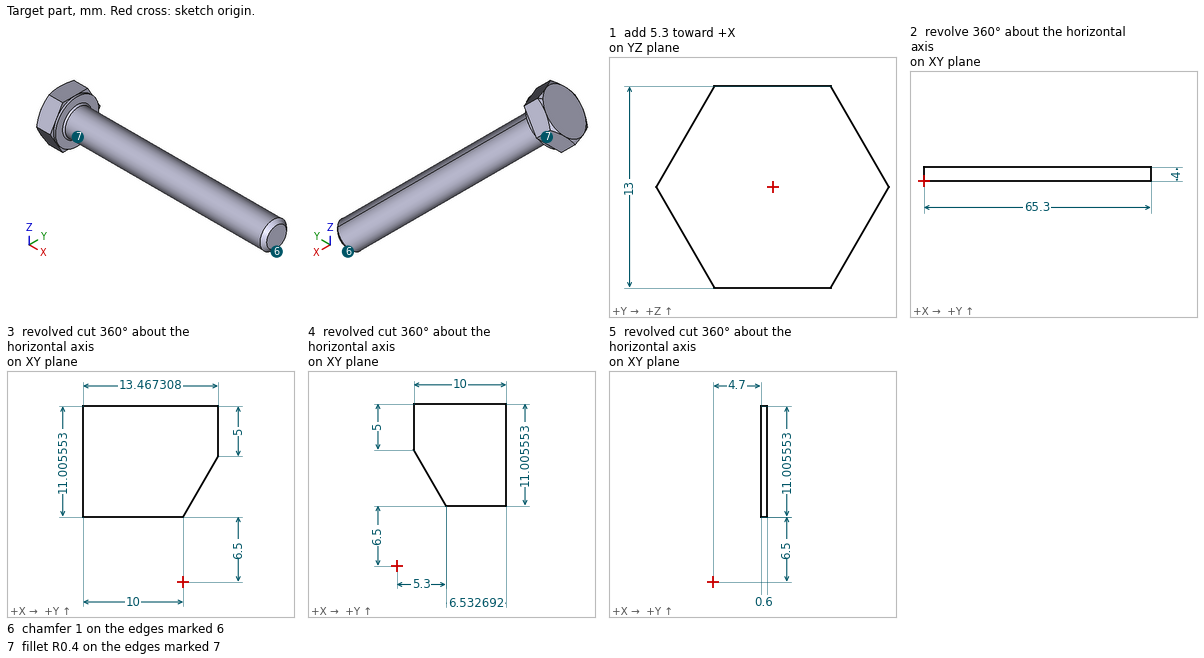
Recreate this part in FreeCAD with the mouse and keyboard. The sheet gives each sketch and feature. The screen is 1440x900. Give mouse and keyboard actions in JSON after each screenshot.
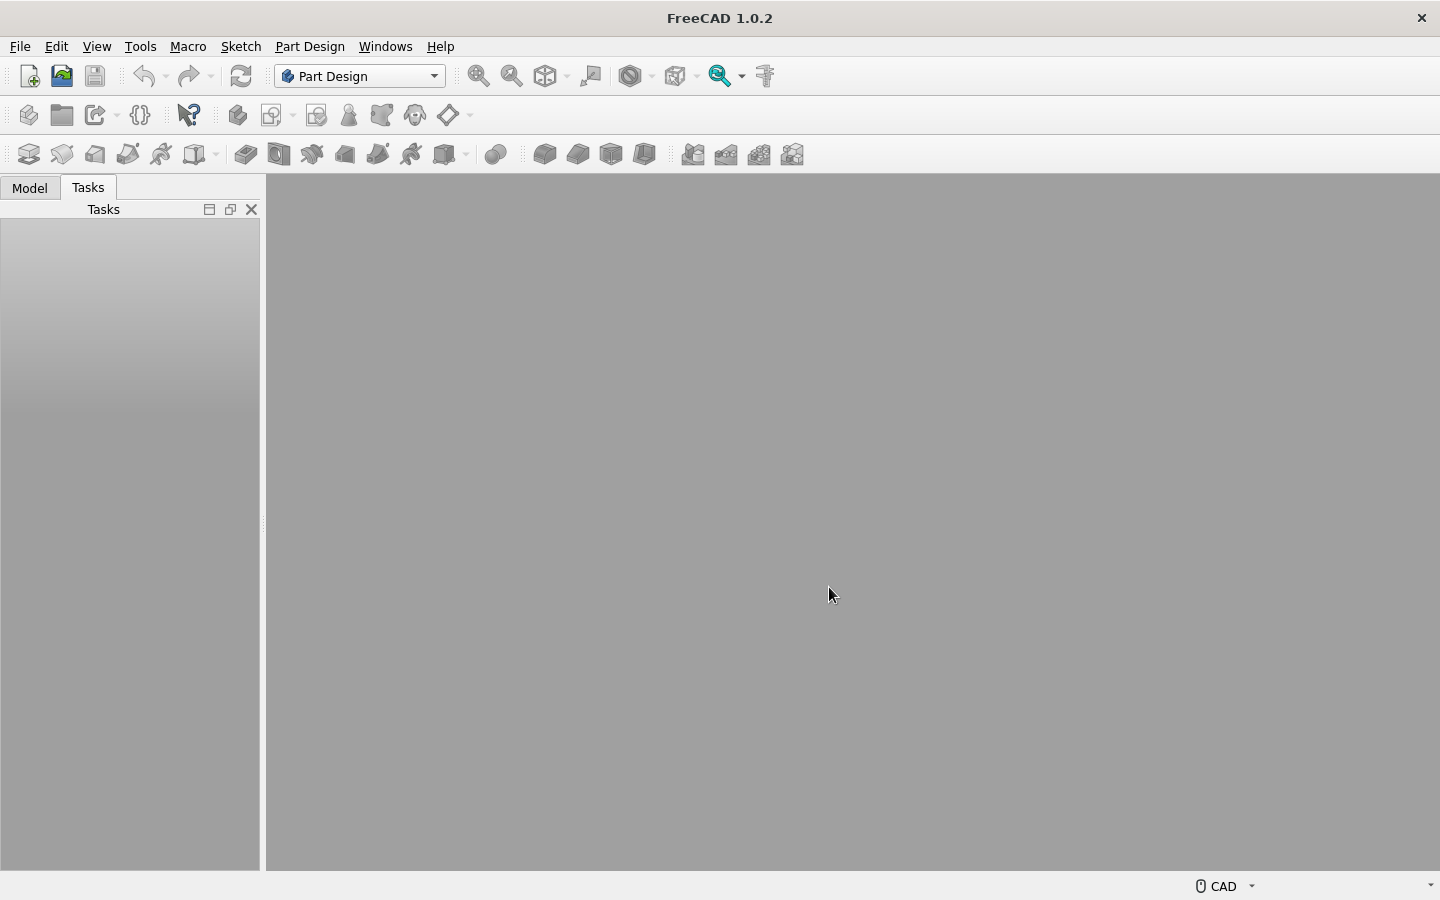
{"action": "left_click", "coordinate": [29, 76]}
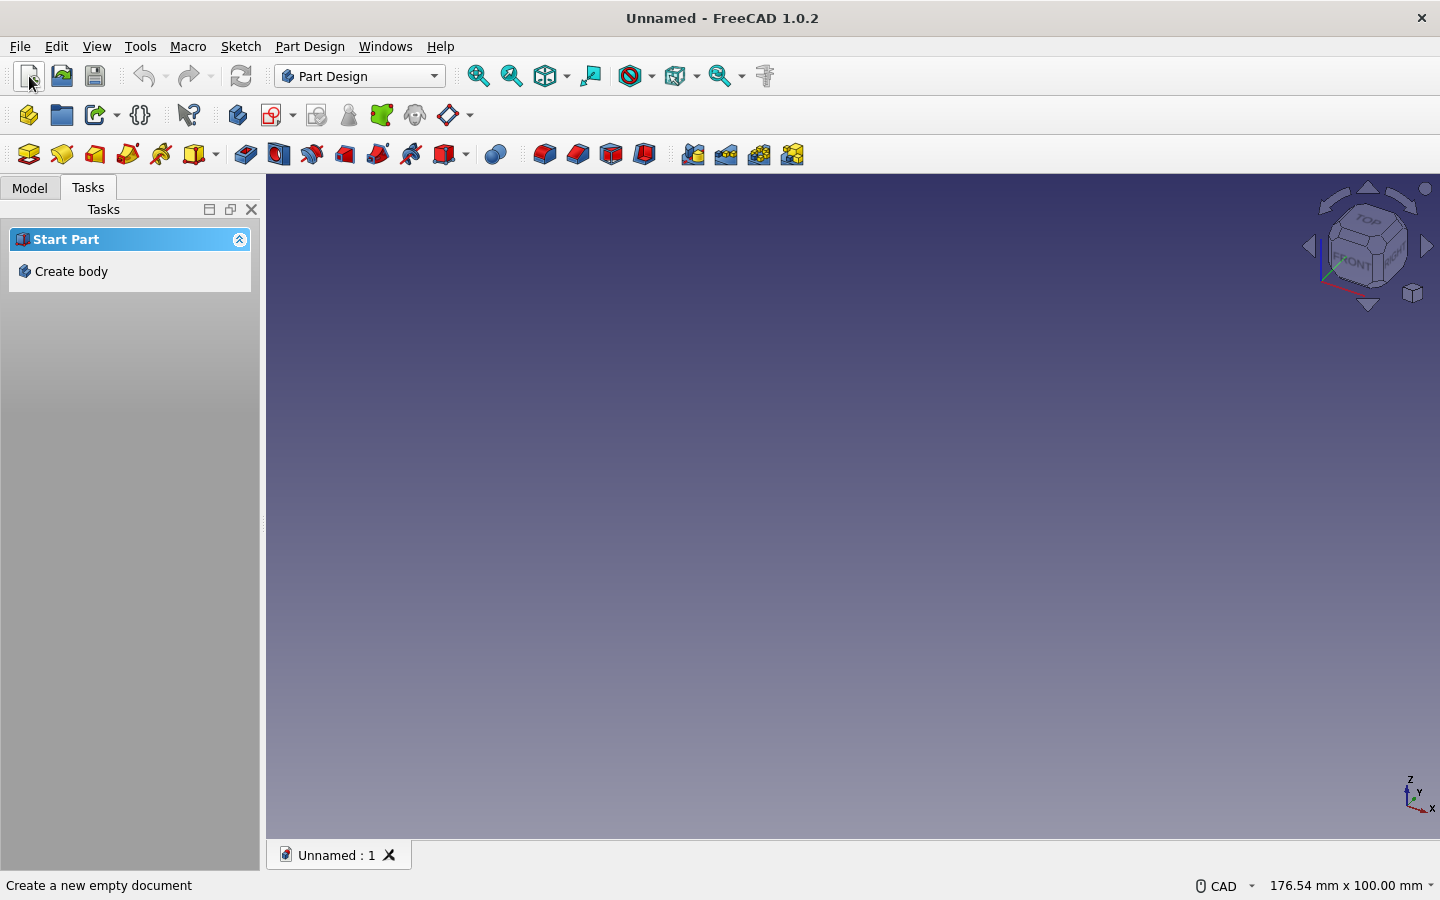
{"action": "left_click", "coordinate": [270, 116]}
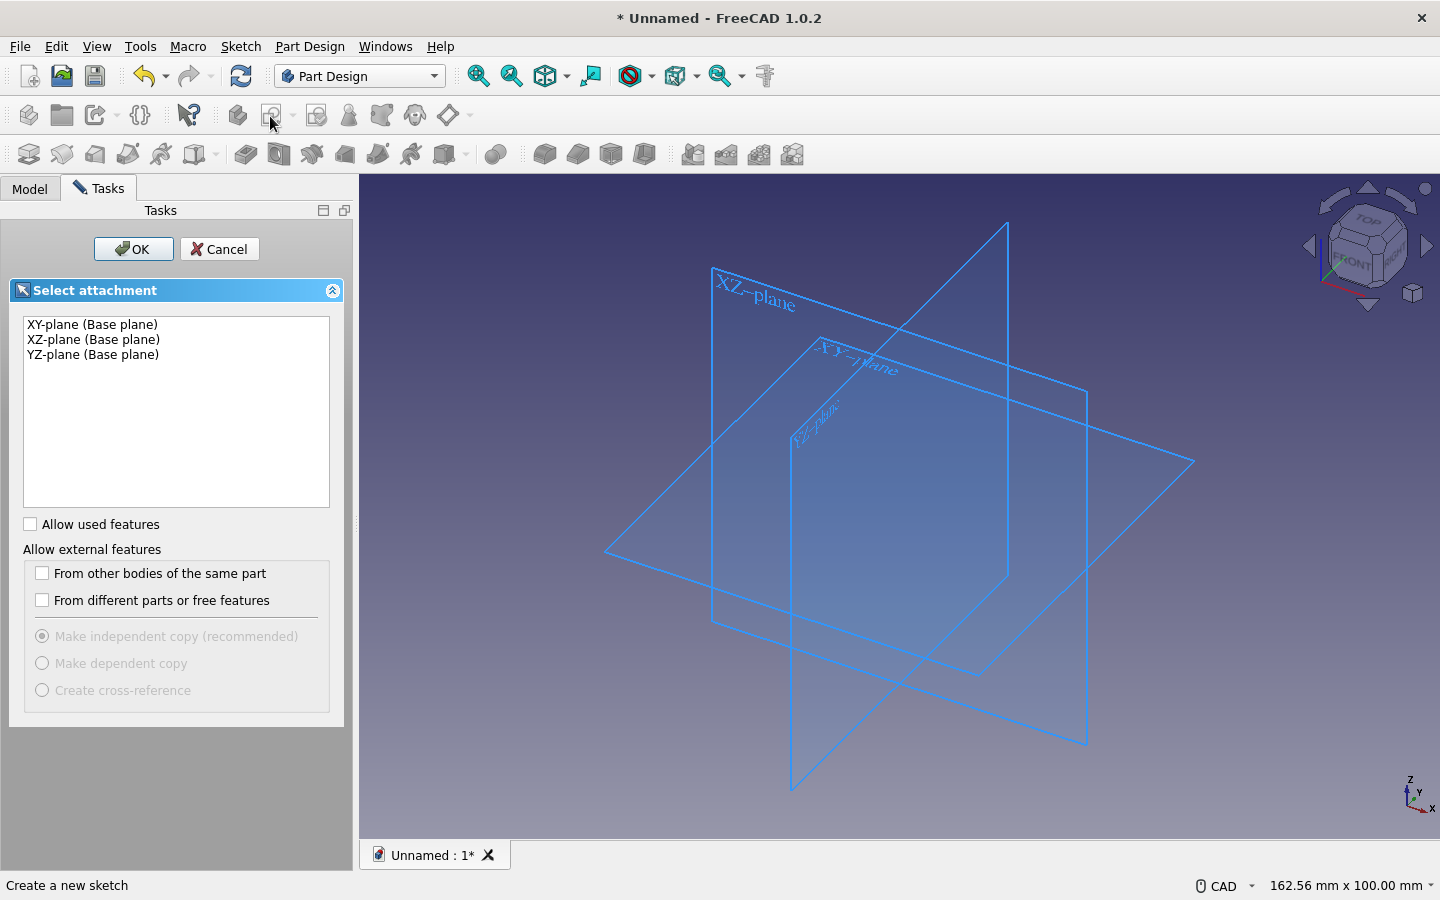
{"action": "left_click", "coordinate": [84, 354]}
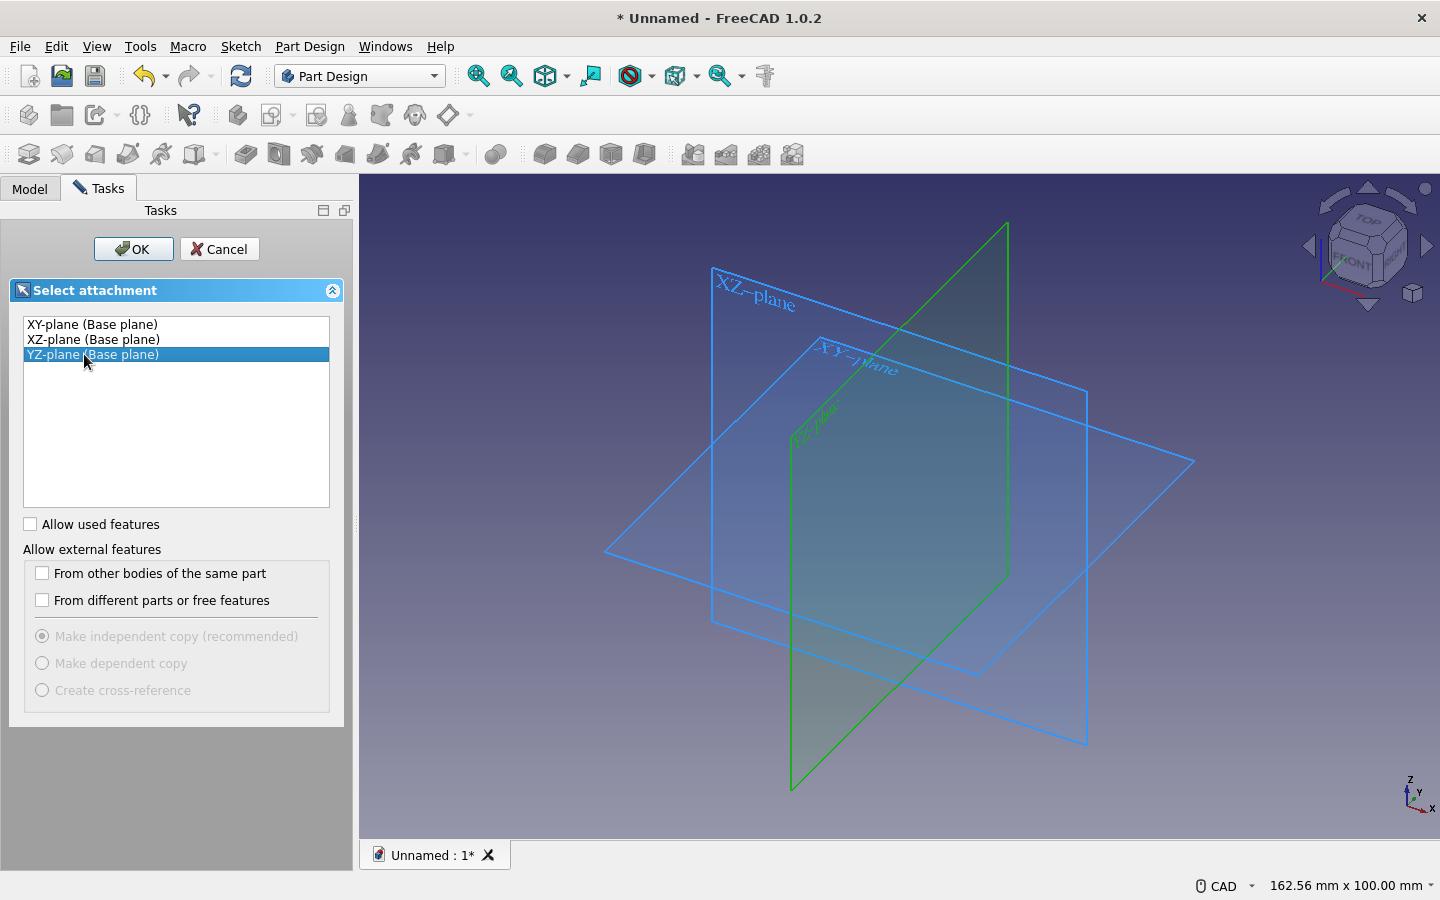
{"action": "left_click", "coordinate": [134, 249]}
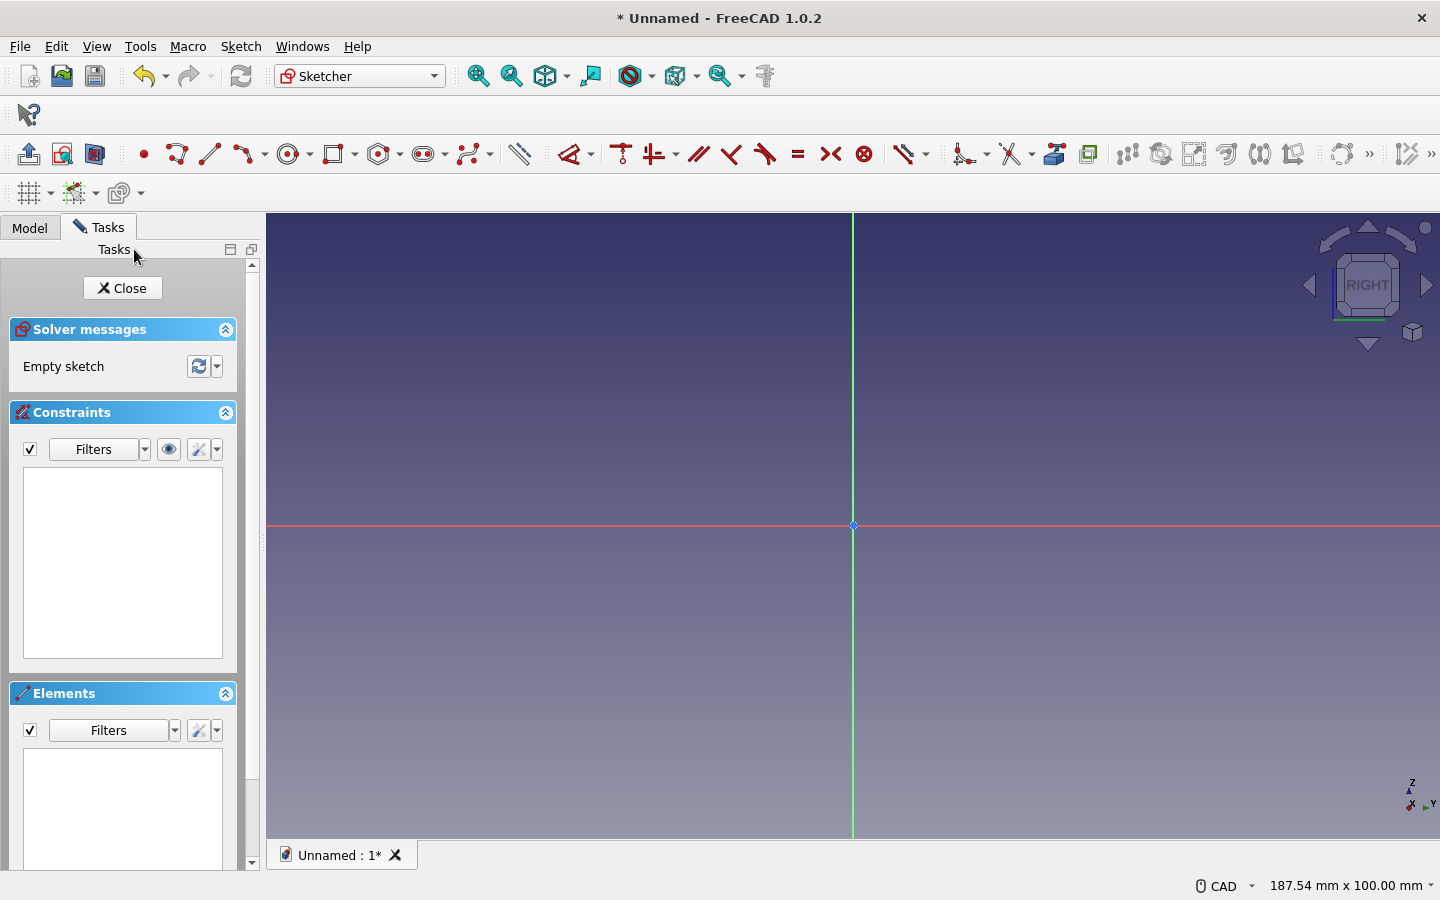
{"action": "scroll", "coordinate": [870, 526], "scroll_direction": "up", "scroll_amount": 8}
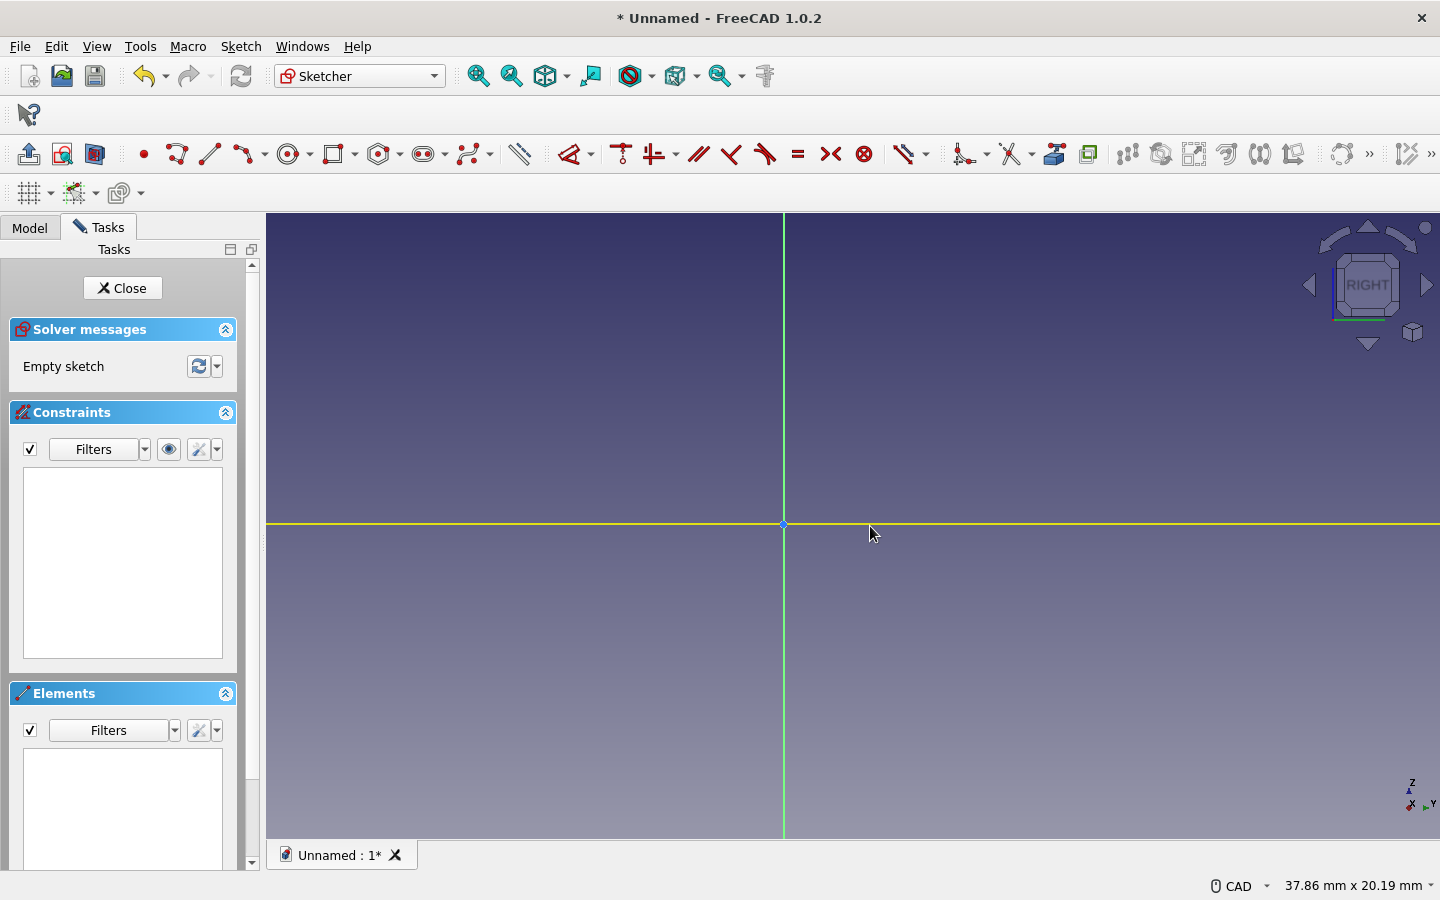
{"action": "left_click", "coordinate": [378, 154]}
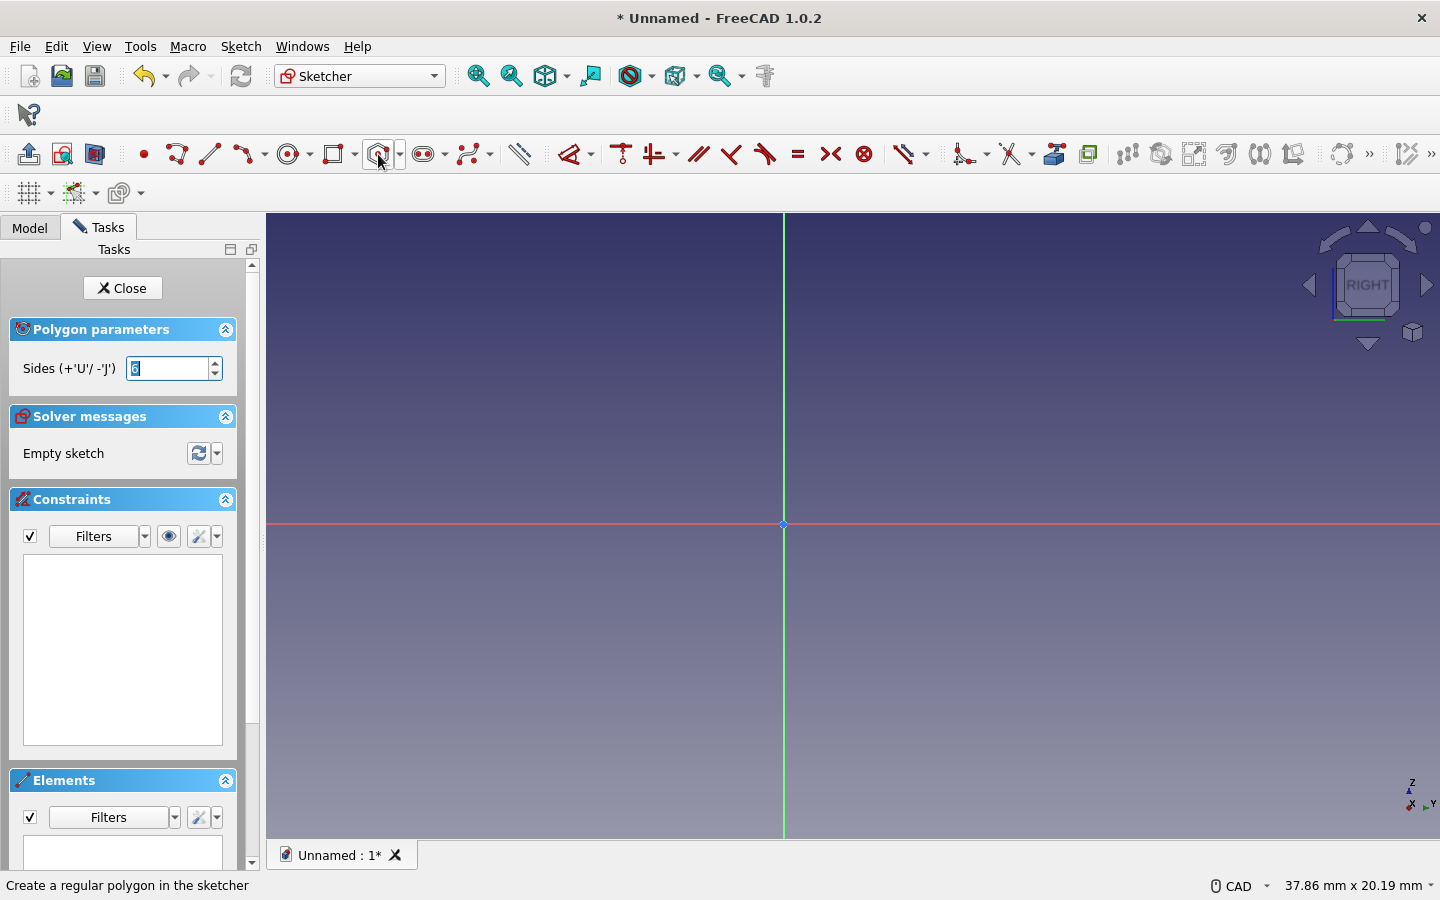
{"action": "left_click", "coordinate": [784, 524]}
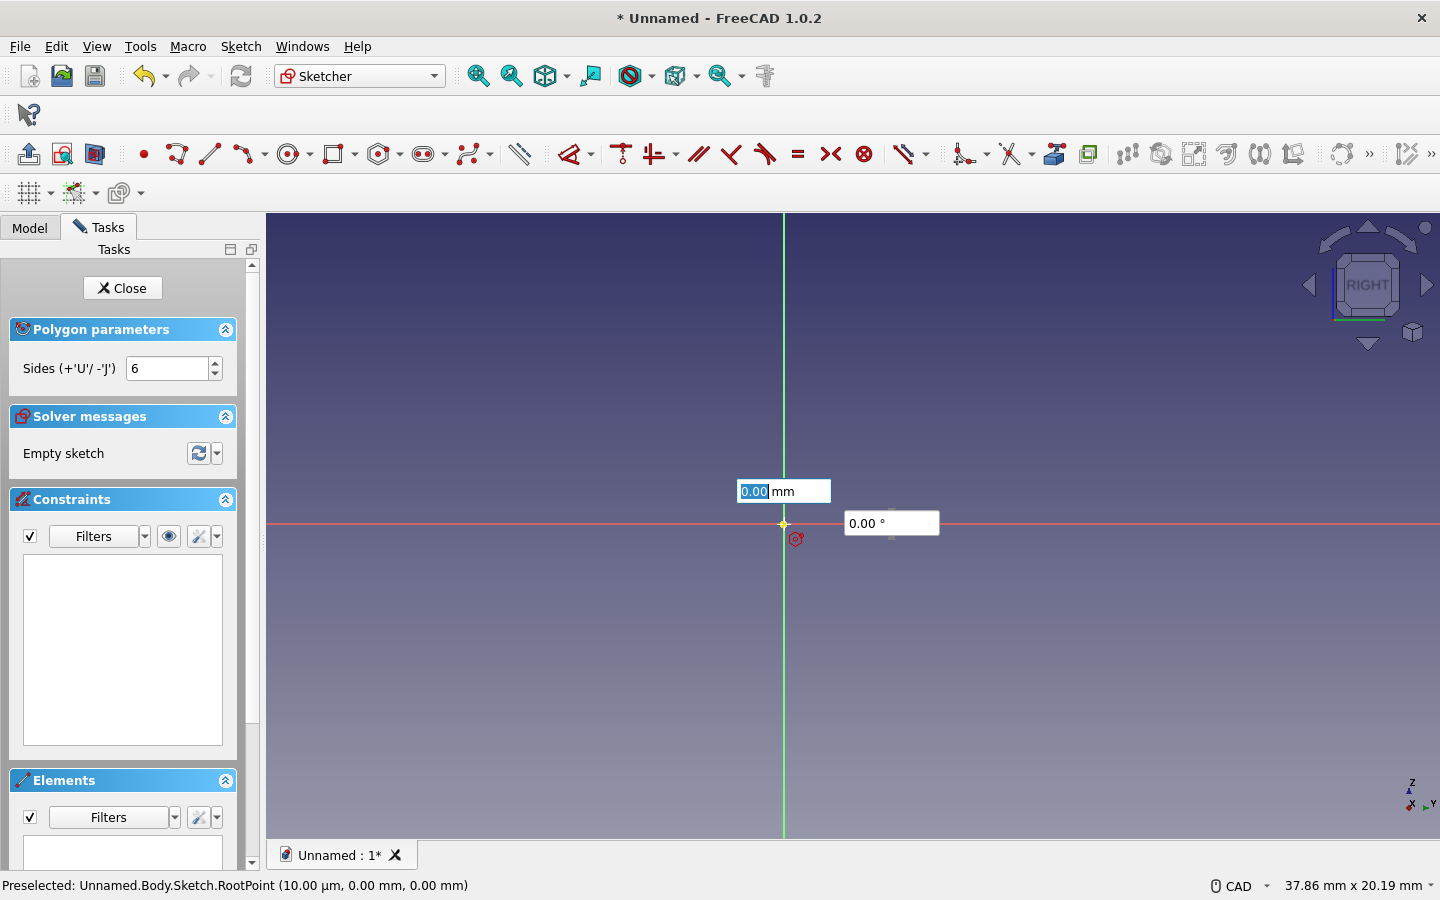
{"action": "left_click", "coordinate": [1016, 524]}
{"action": "key", "text": "Escape"}